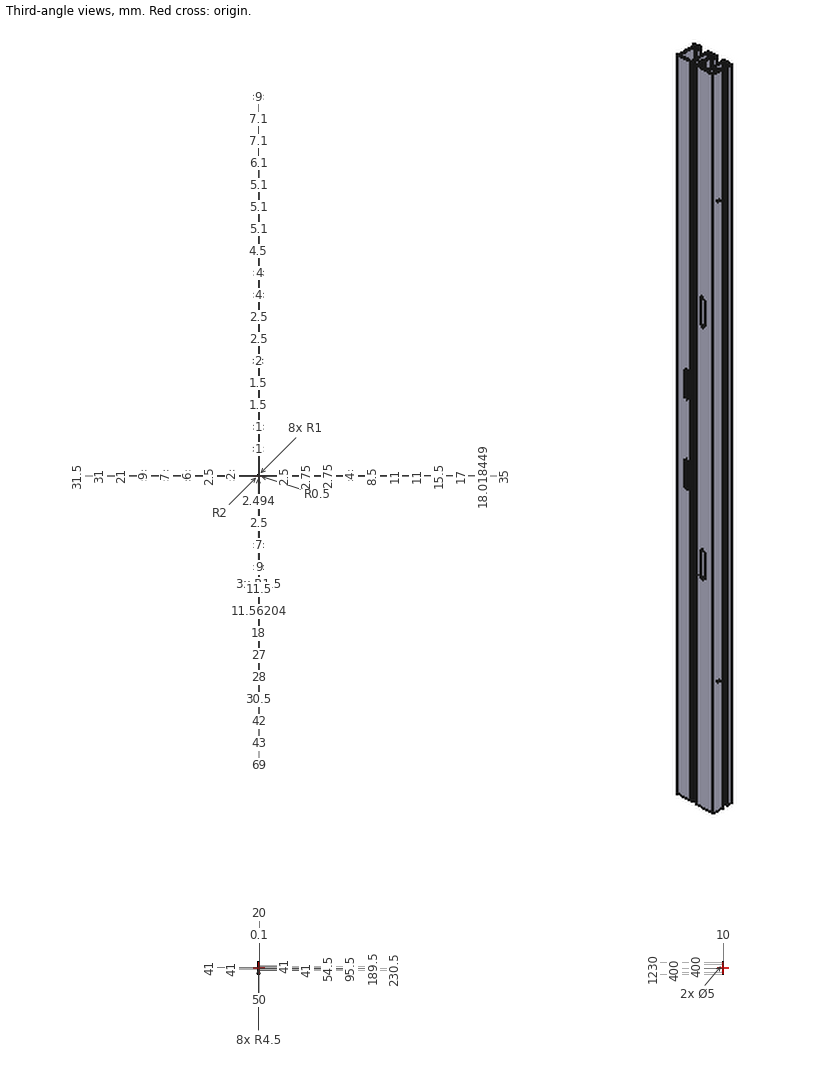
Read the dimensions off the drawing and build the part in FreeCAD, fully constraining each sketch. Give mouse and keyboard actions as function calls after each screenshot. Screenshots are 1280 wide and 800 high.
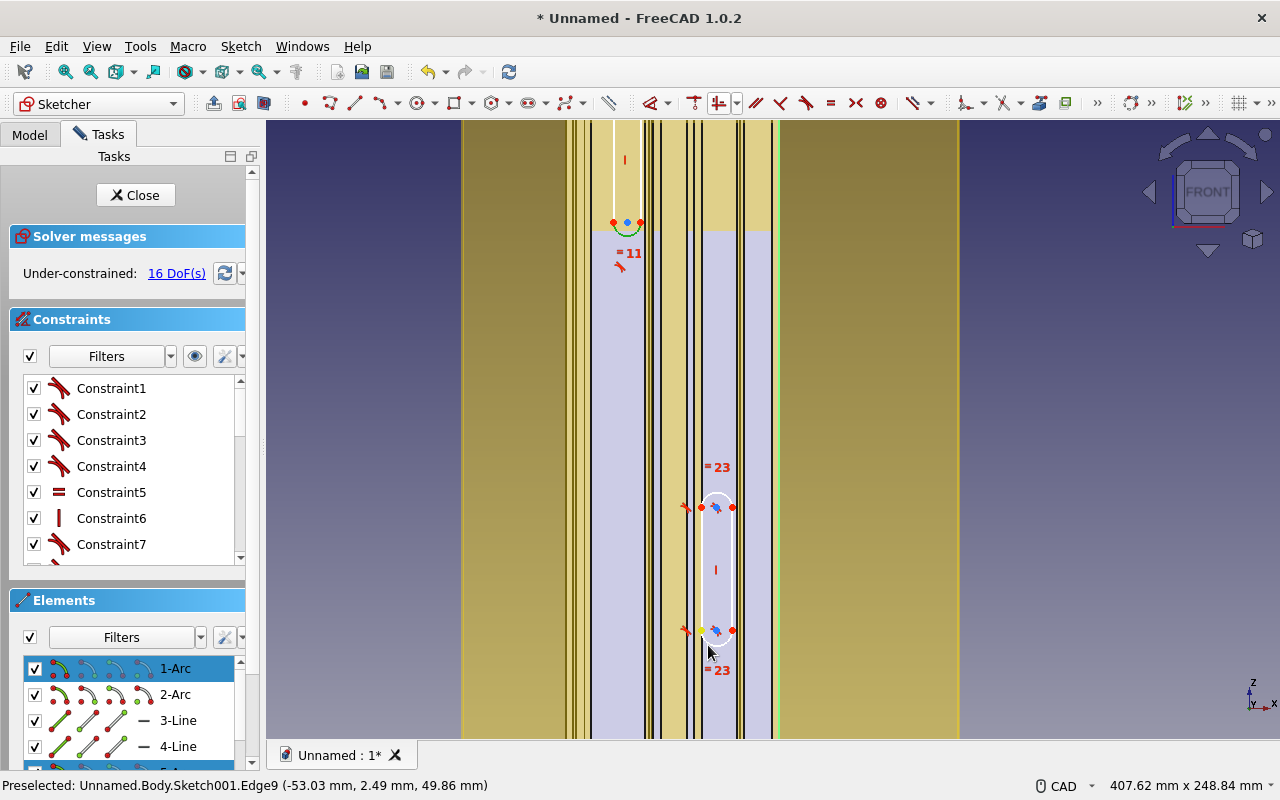
click(708, 643)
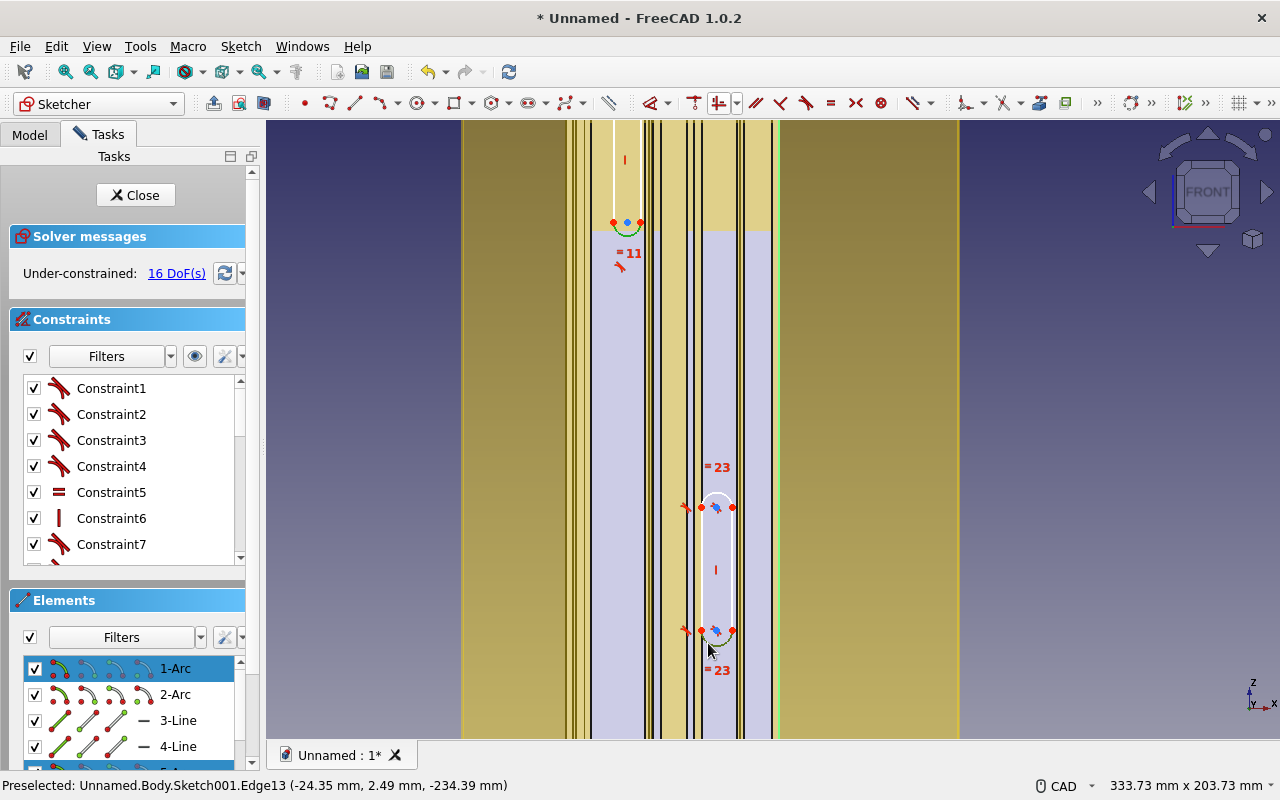
click(831, 104)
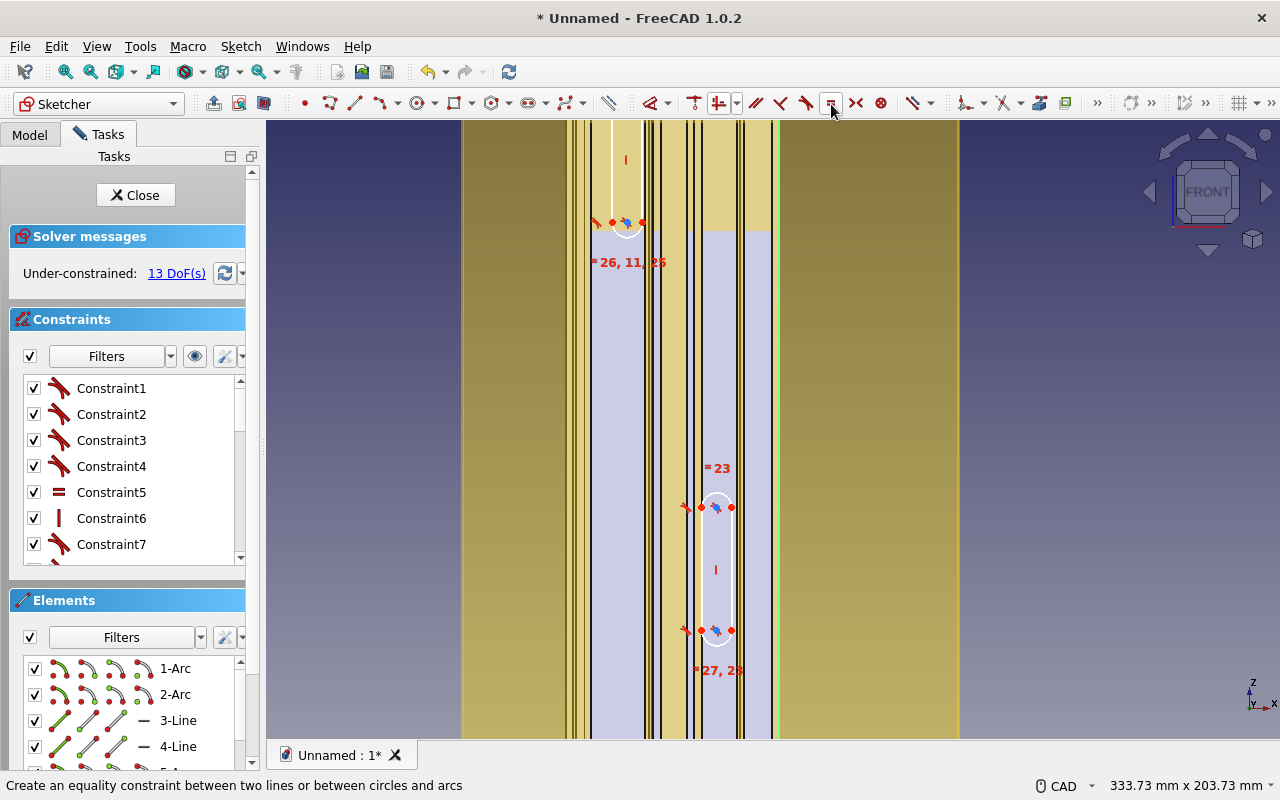
click(650, 104)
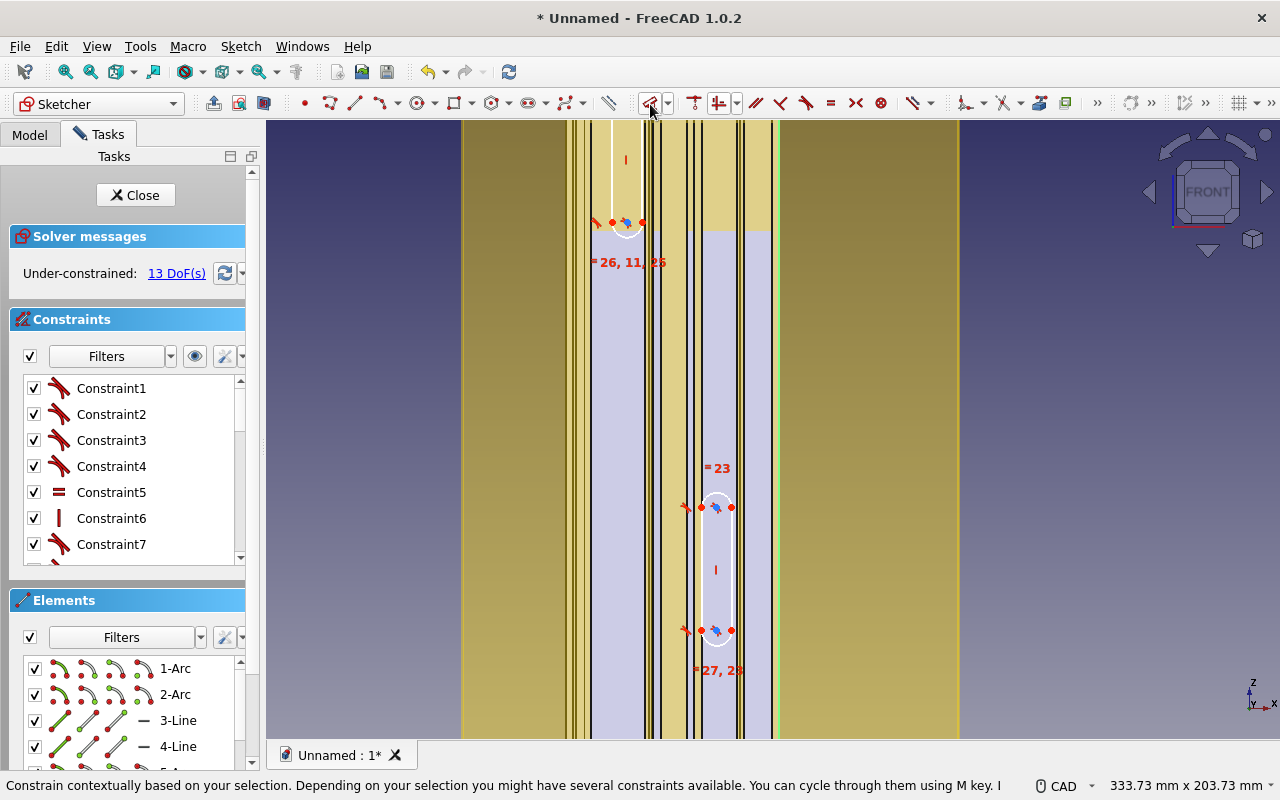
scroll(708, 646, down, 6)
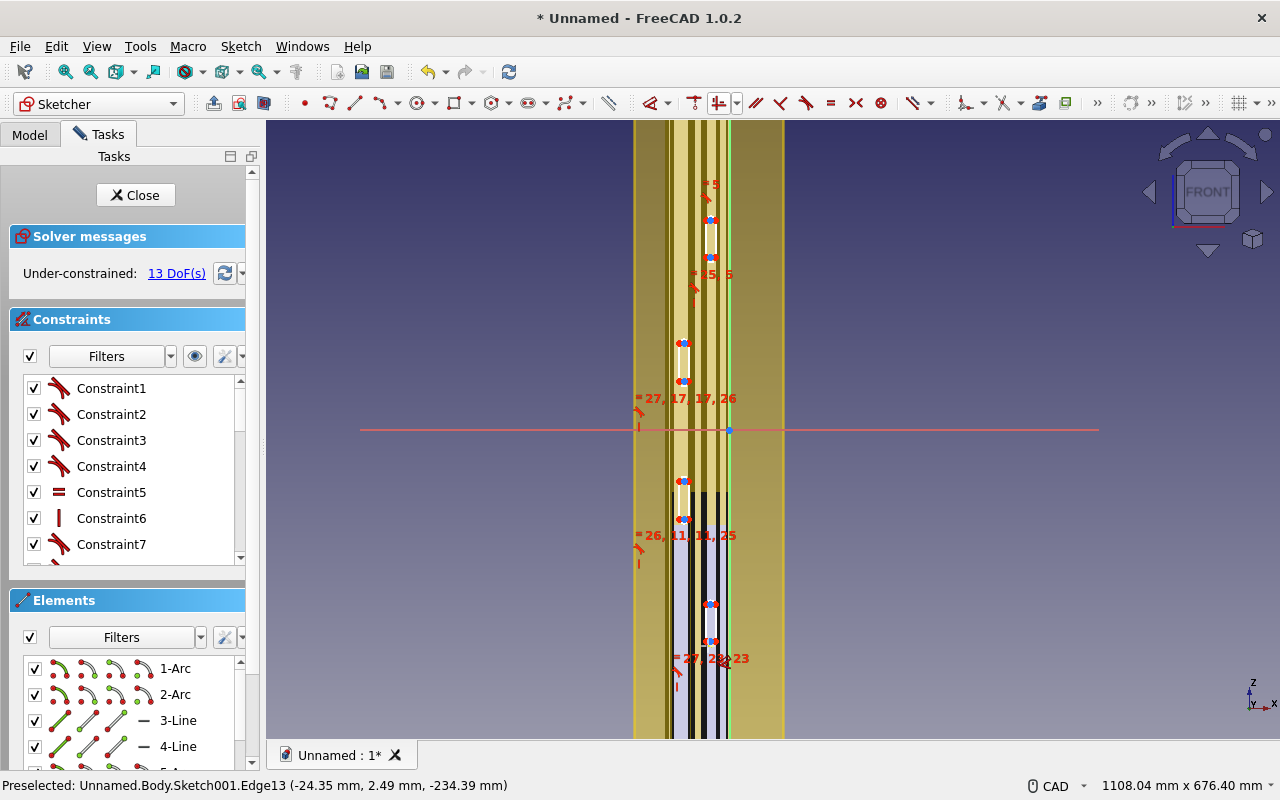
scroll(708, 262, up, 12)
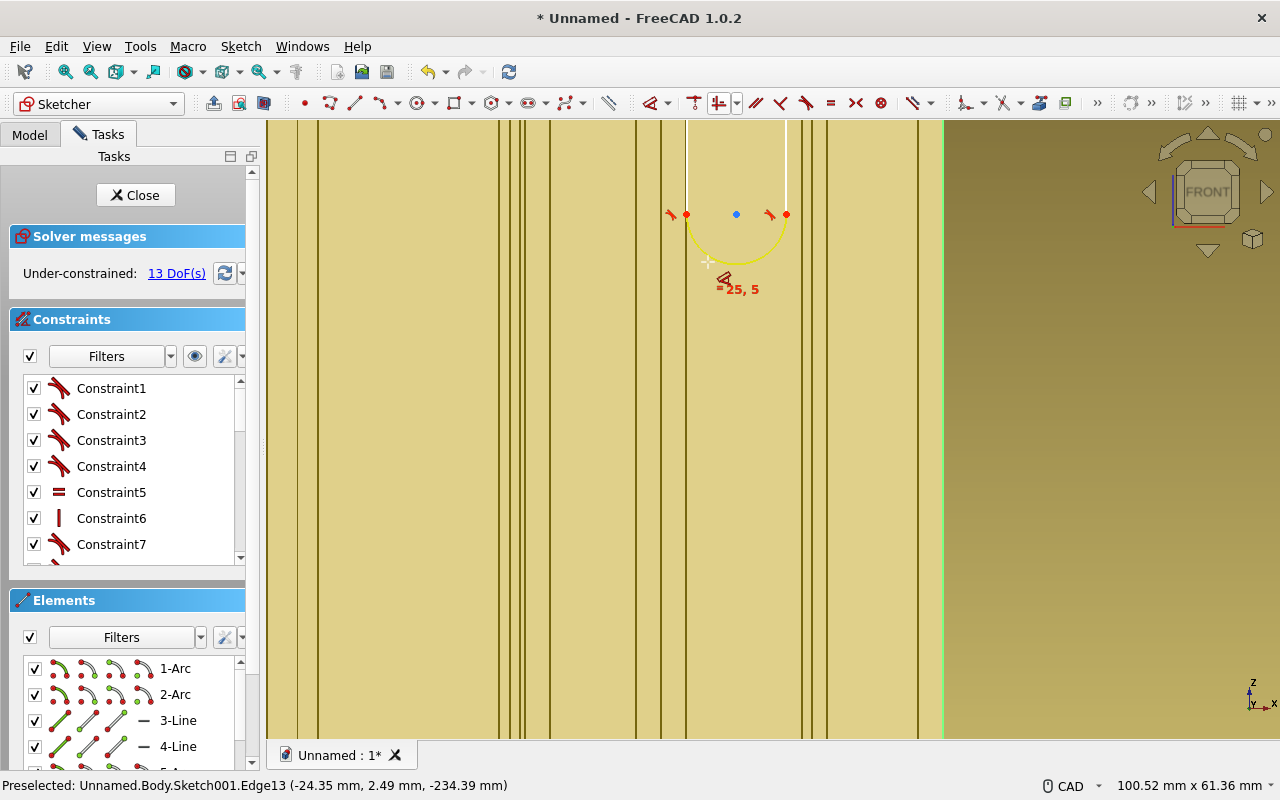
click(707, 255)
click(688, 281)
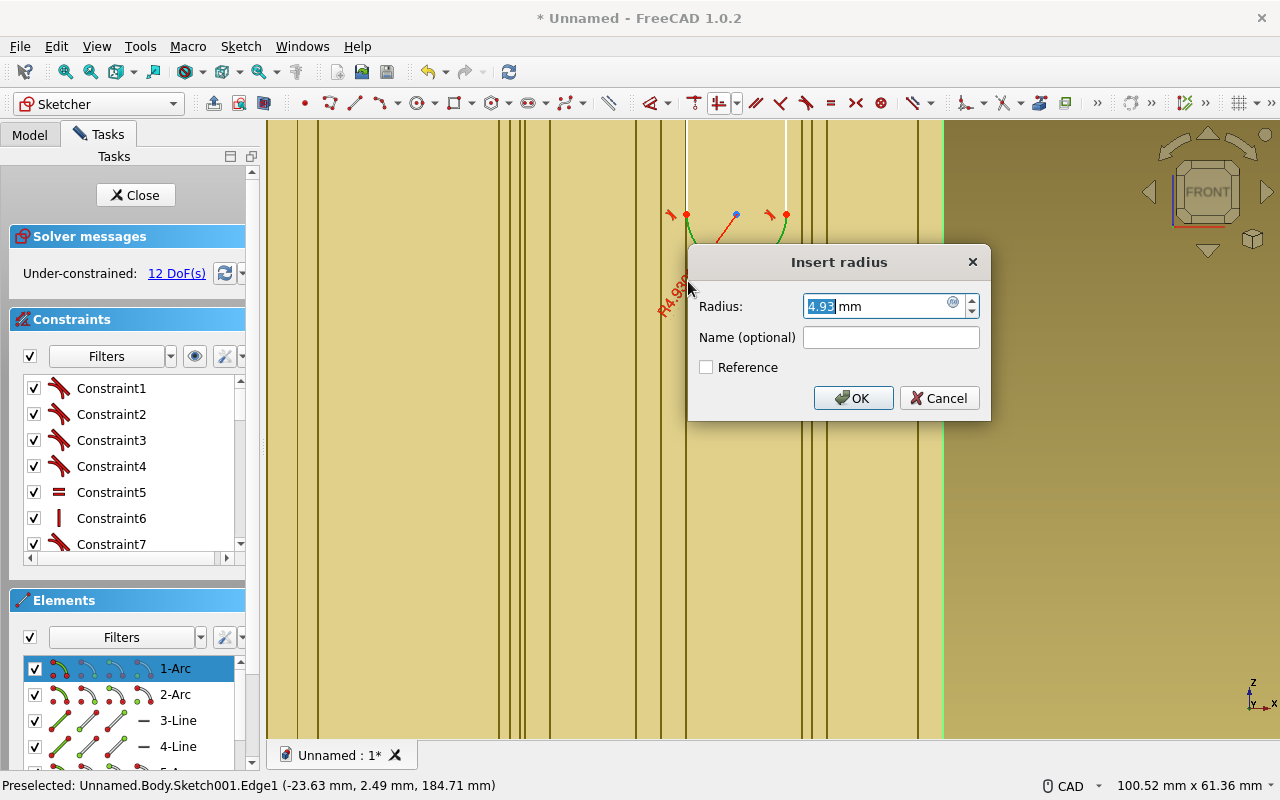
text(4.5)
key(Return)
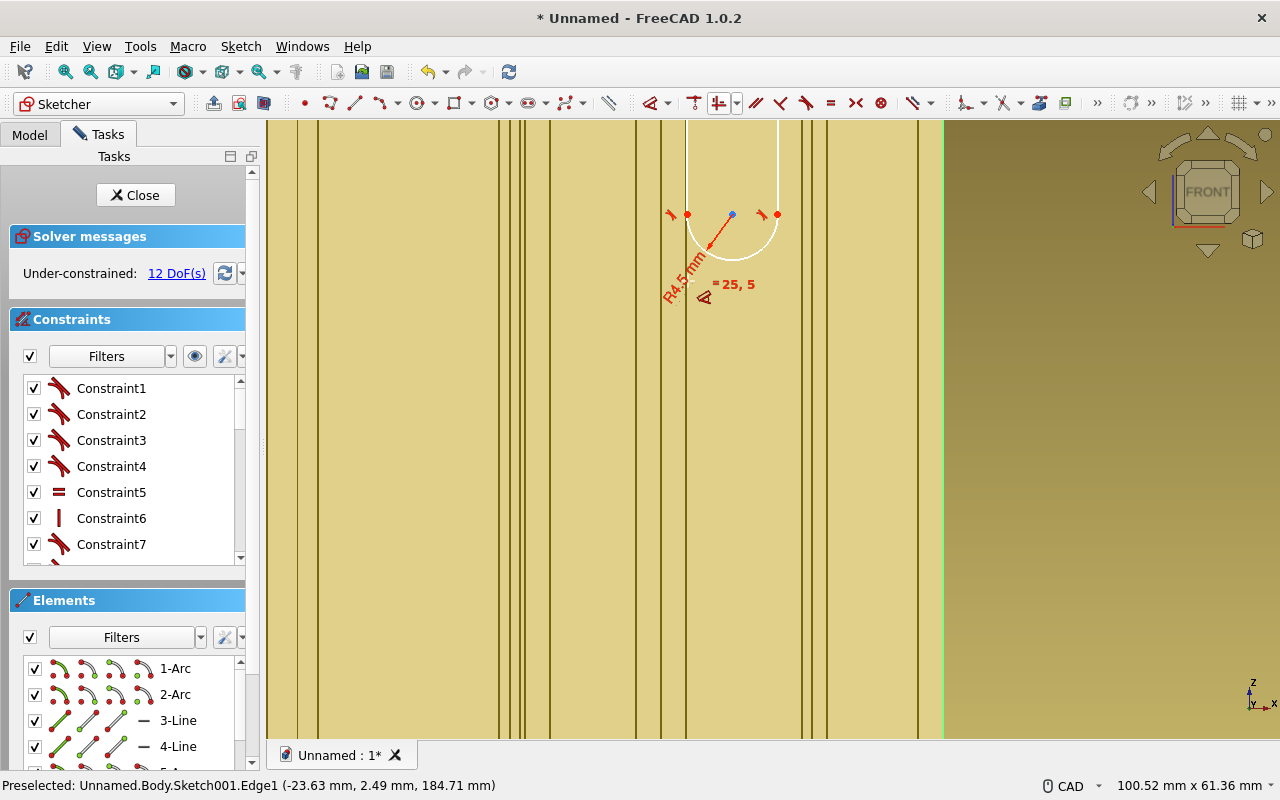
scroll(708, 261, down, 12)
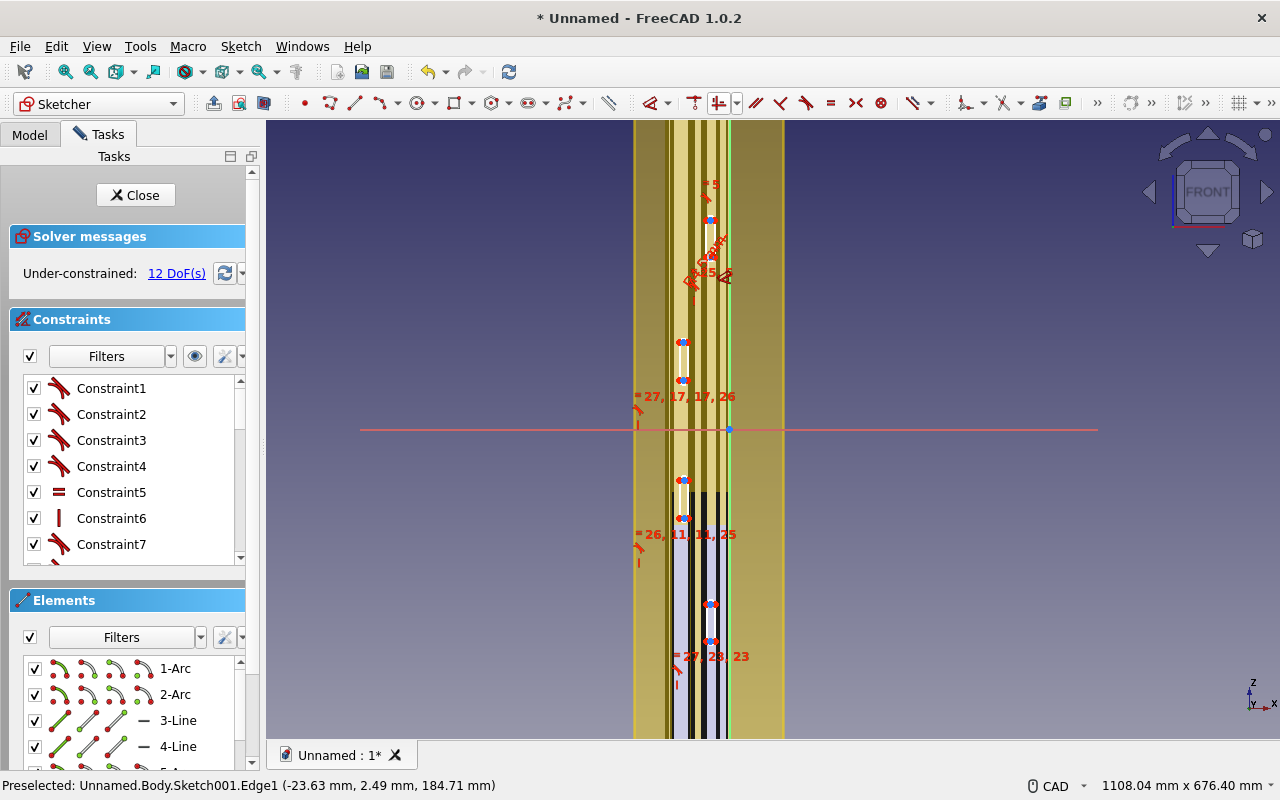
scroll(706, 246, up, 3)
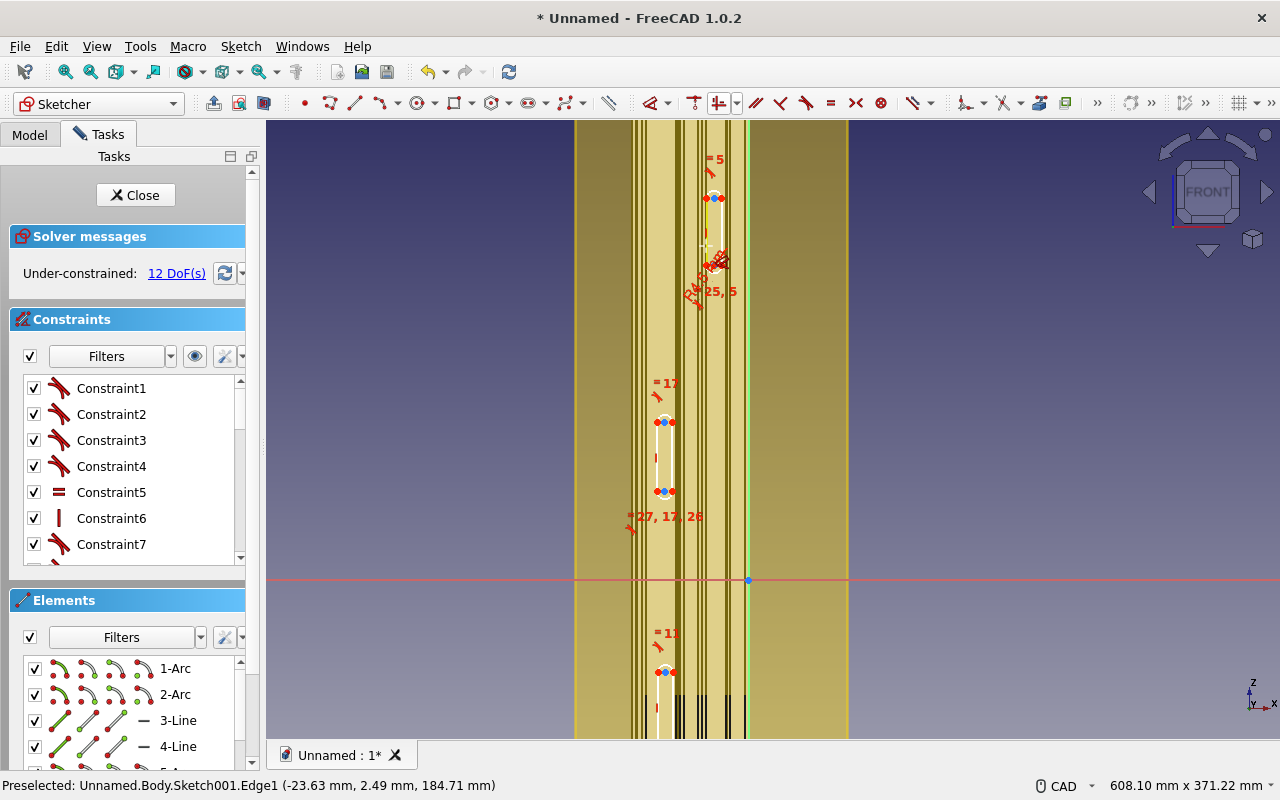
click(707, 246)
click(673, 232)